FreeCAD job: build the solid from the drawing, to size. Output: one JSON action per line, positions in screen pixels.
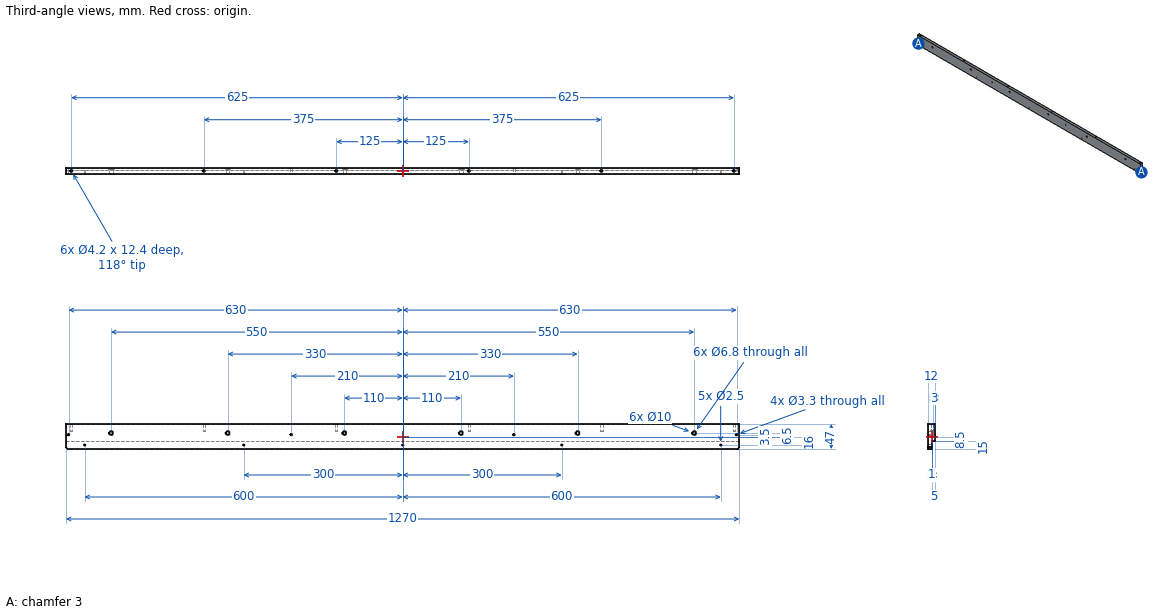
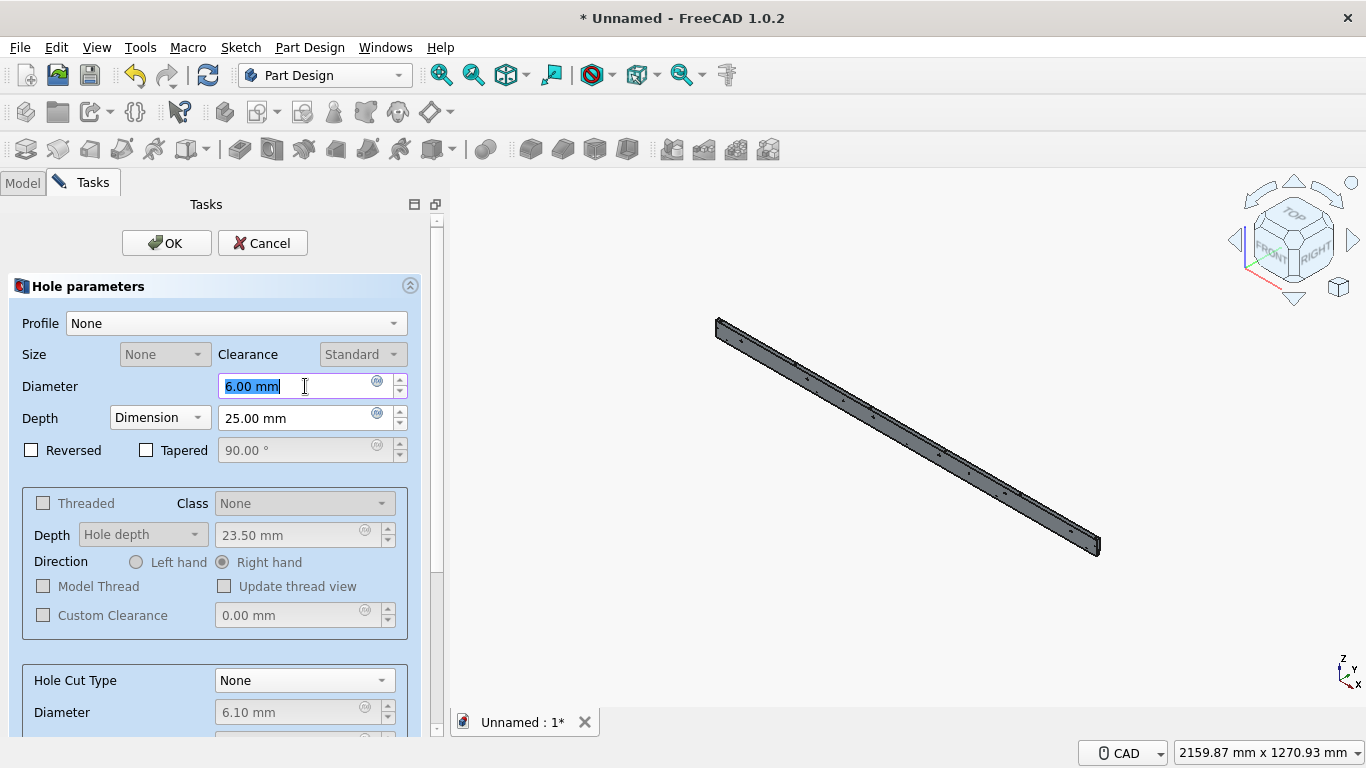
{"action": "type", "text": "6.8"}
{"action": "key", "text": "Tab"}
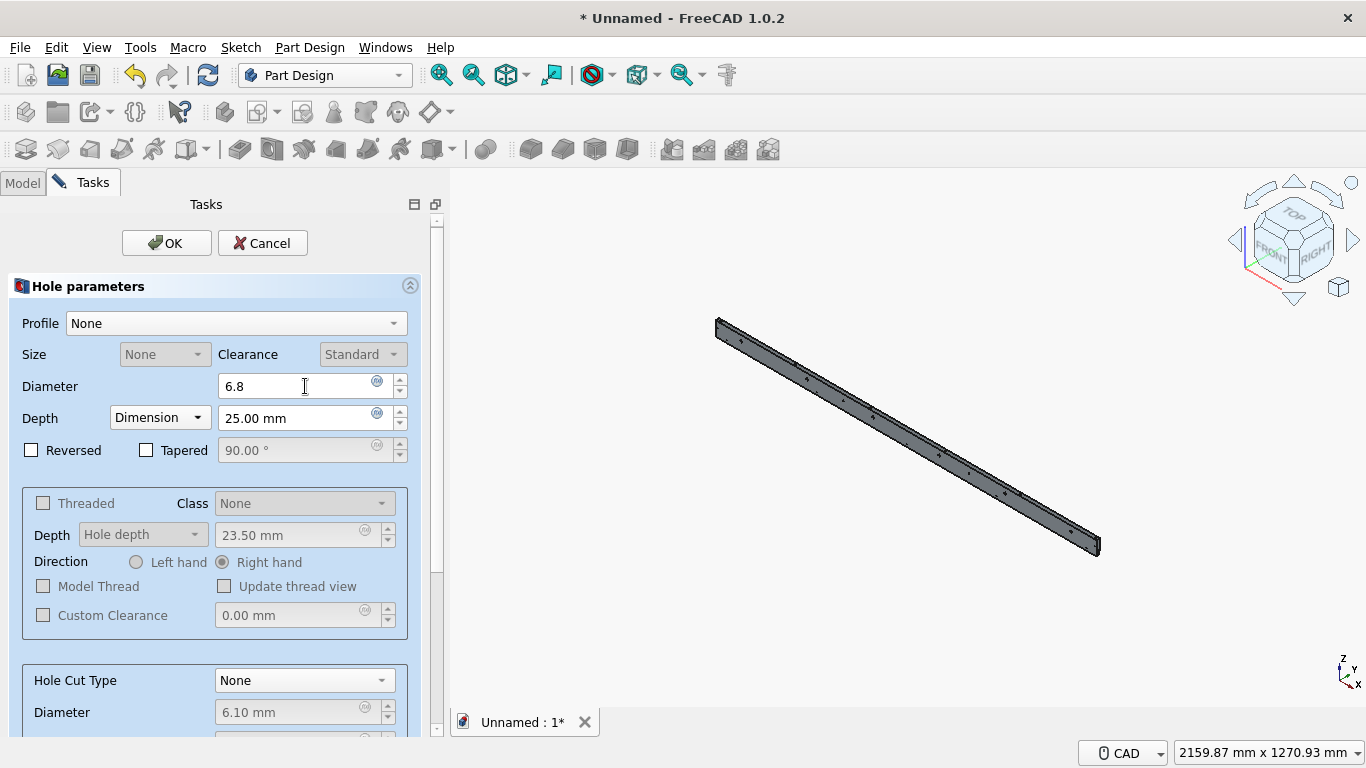
{"action": "left_click", "coordinate": [161, 418]}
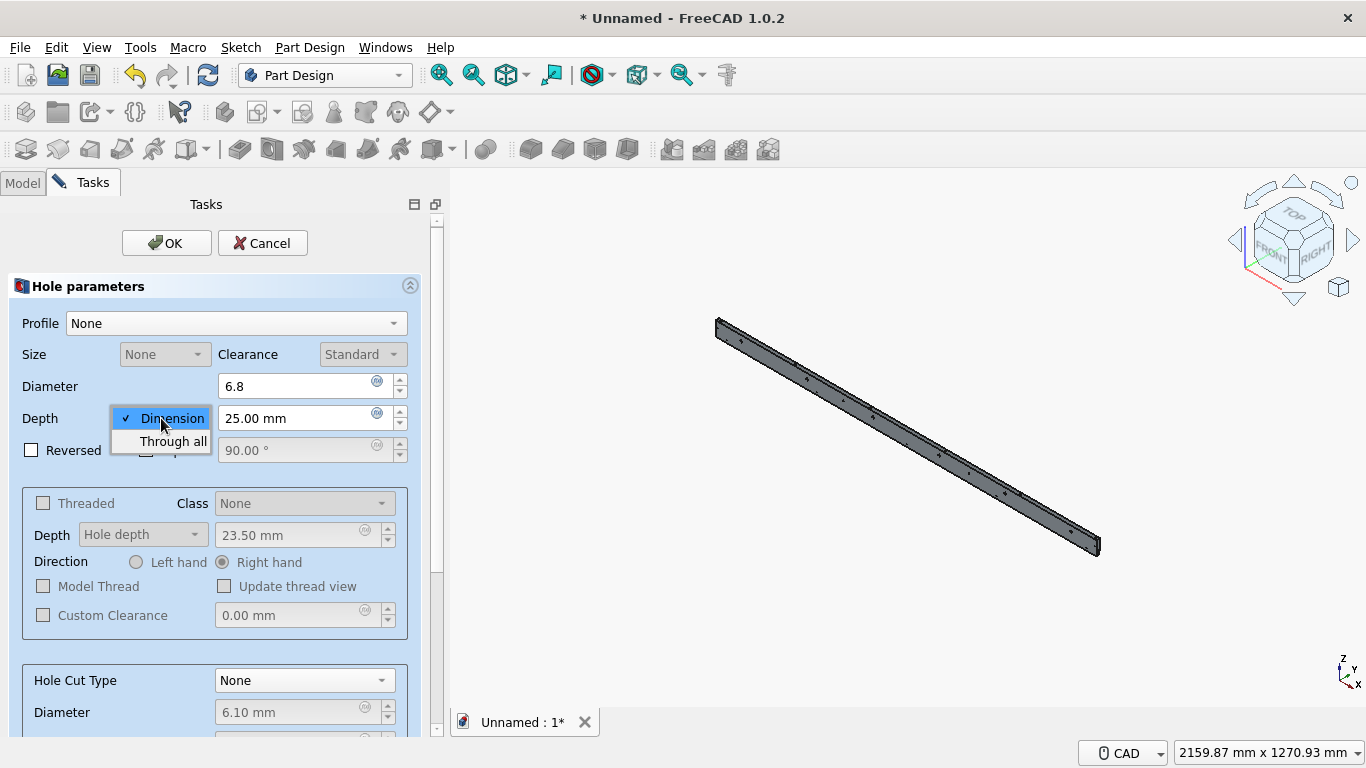
{"action": "left_click", "coordinate": [160, 442]}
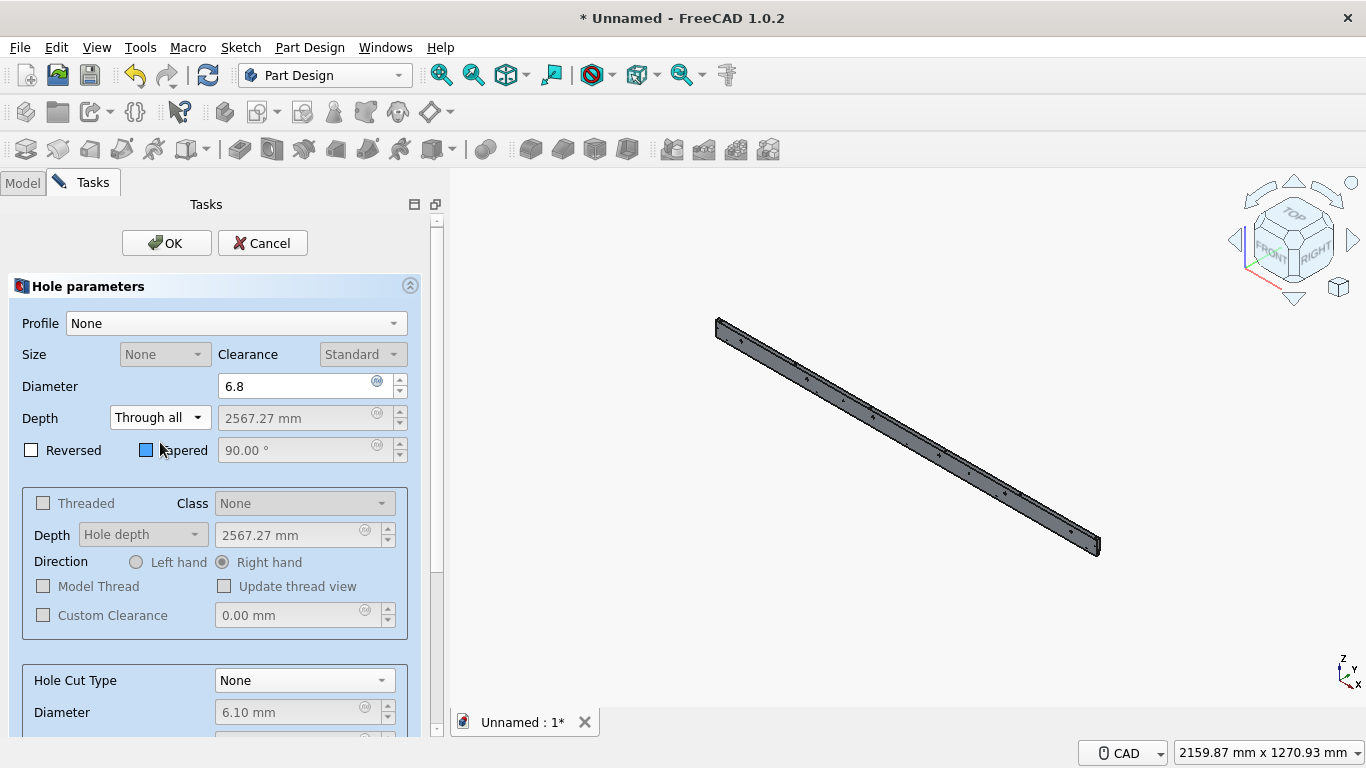
{"action": "left_click", "coordinate": [167, 243]}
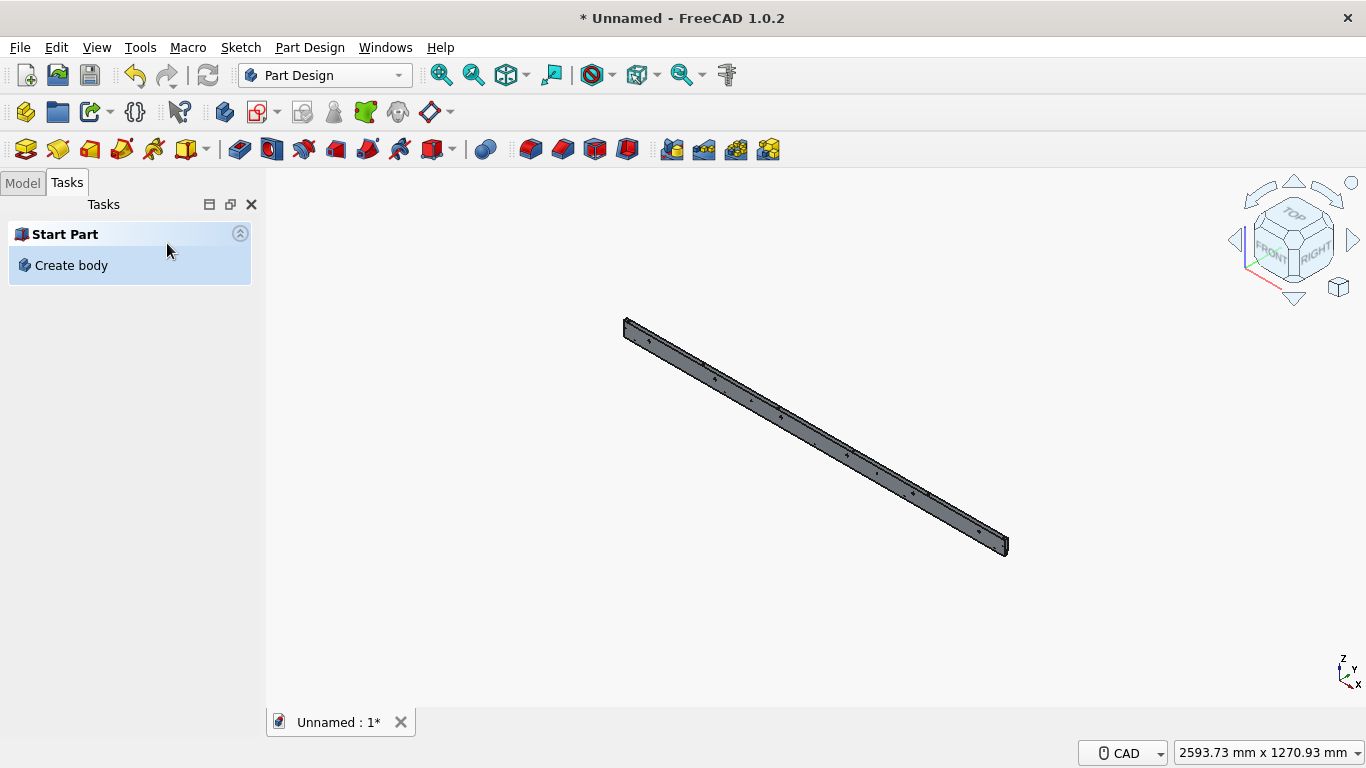
{"action": "left_click", "coordinate": [442, 76]}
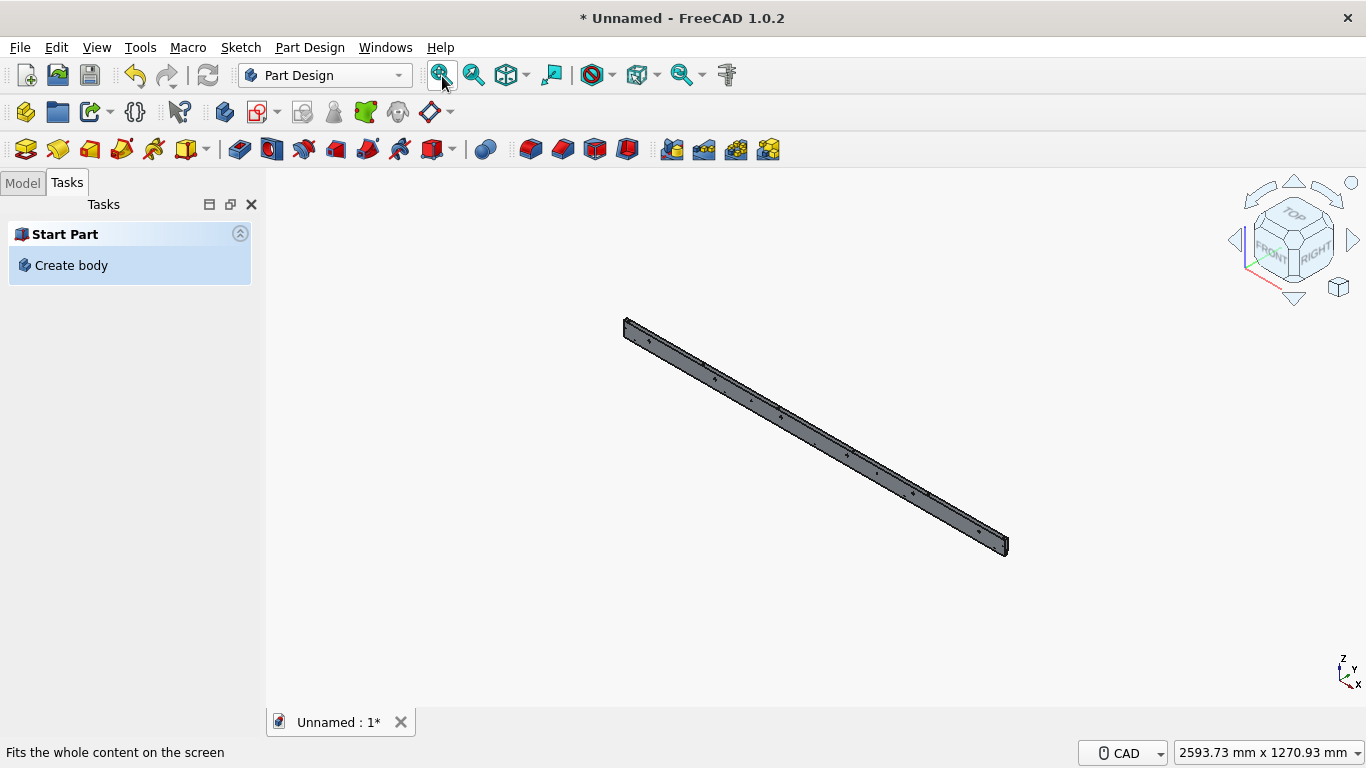
{"action": "key", "text": "4"}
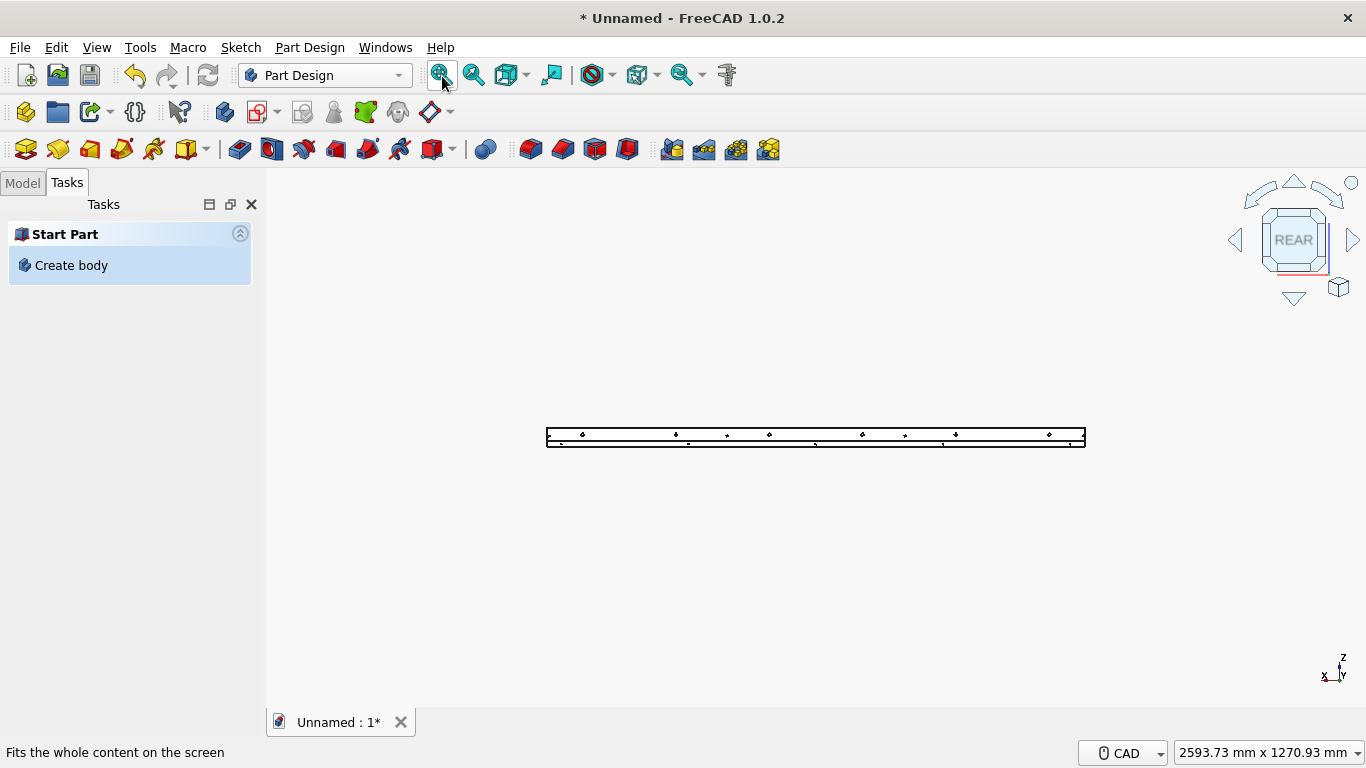
{"action": "left_click", "coordinate": [662, 431]}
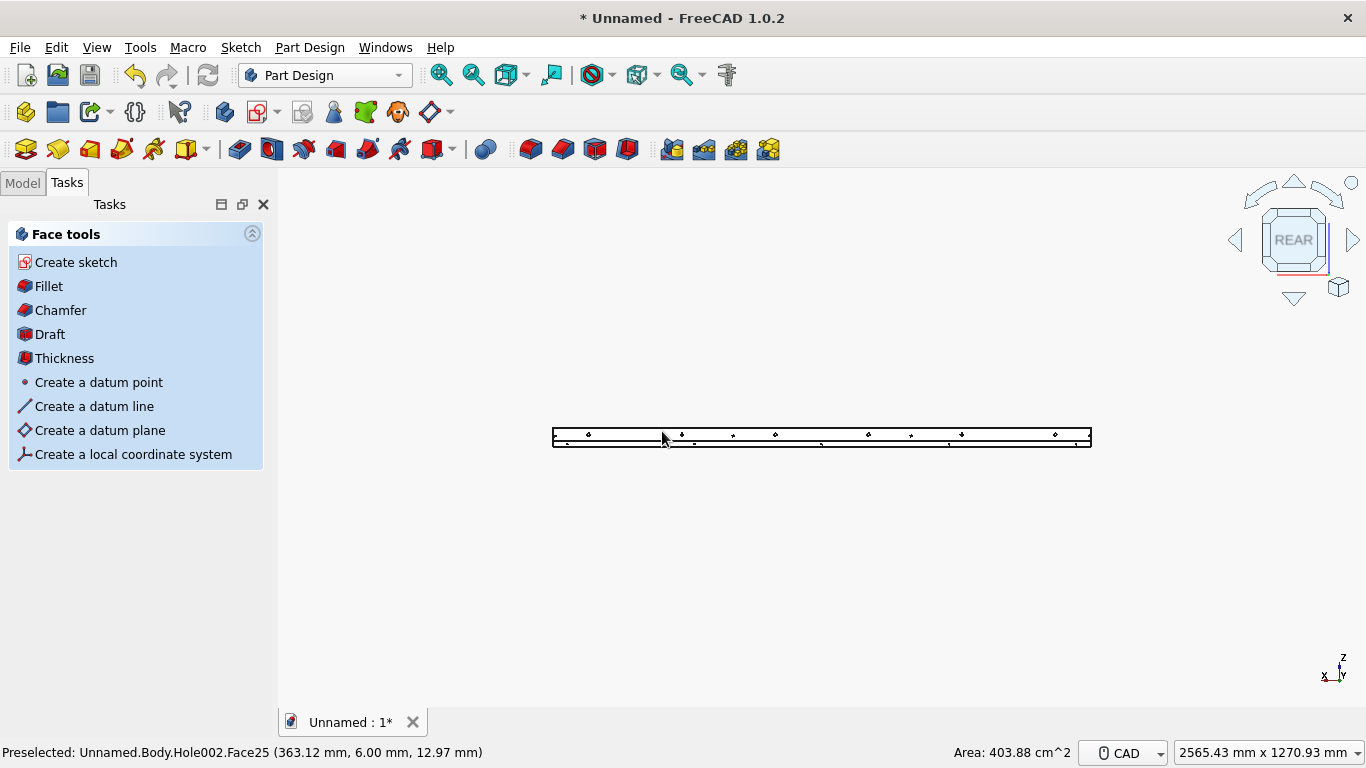
{"action": "left_click", "coordinate": [258, 112]}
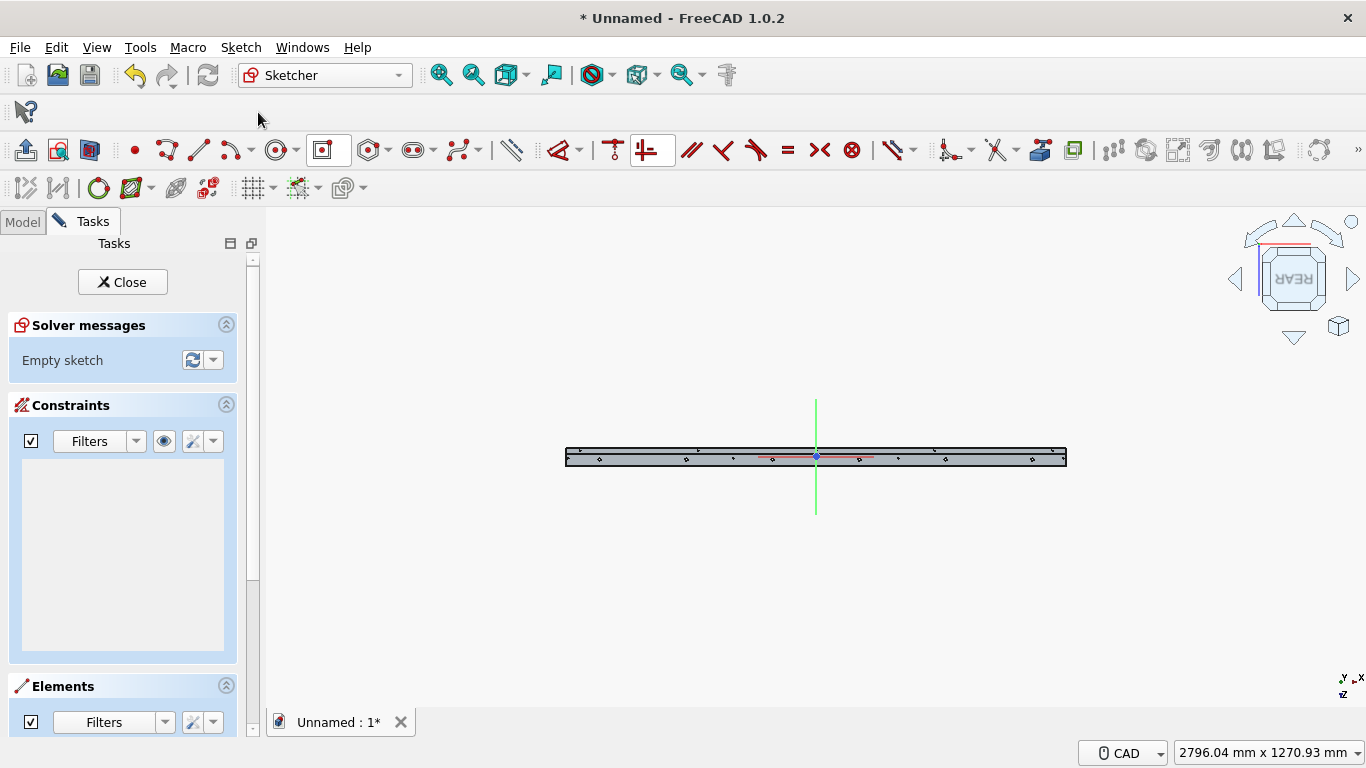
{"action": "scroll", "coordinate": [955, 464], "scroll_direction": "up", "scroll_amount": 2}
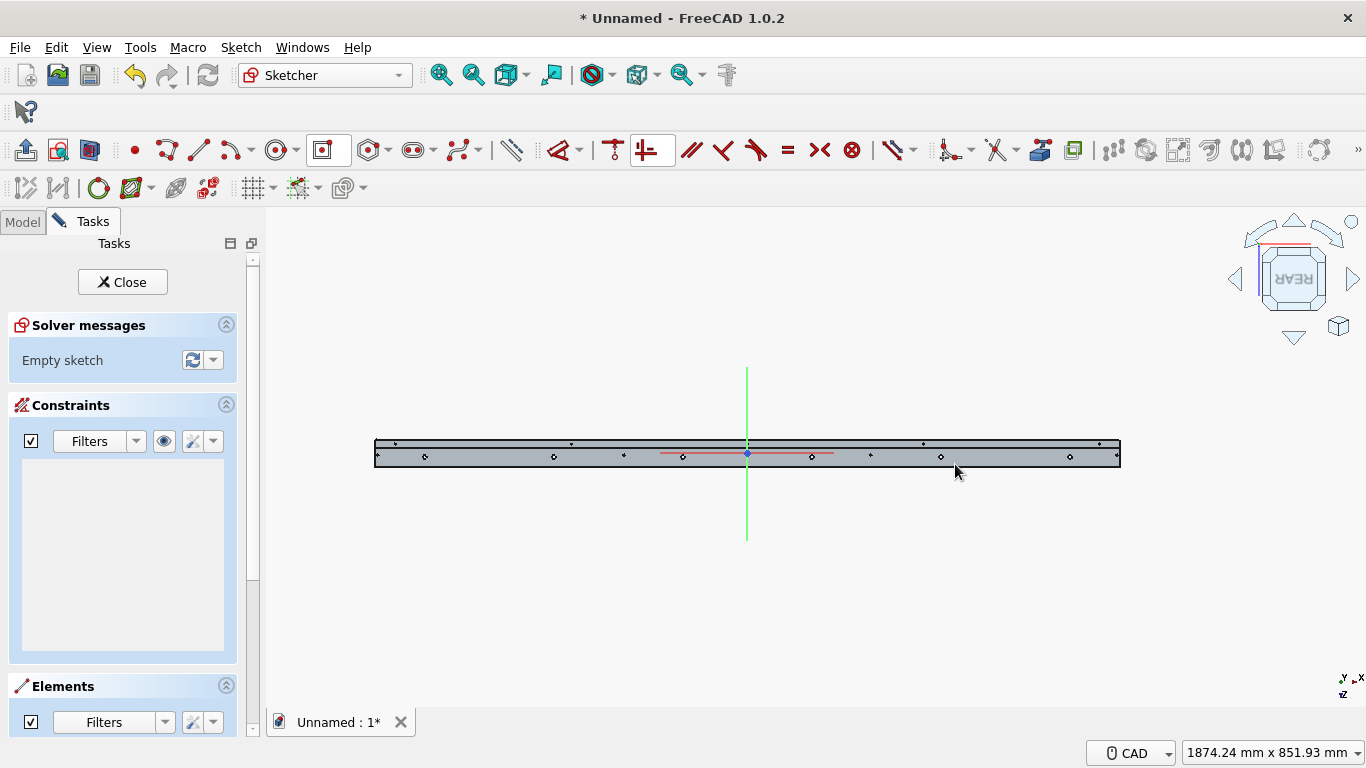
{"action": "left_click", "coordinate": [276, 150]}